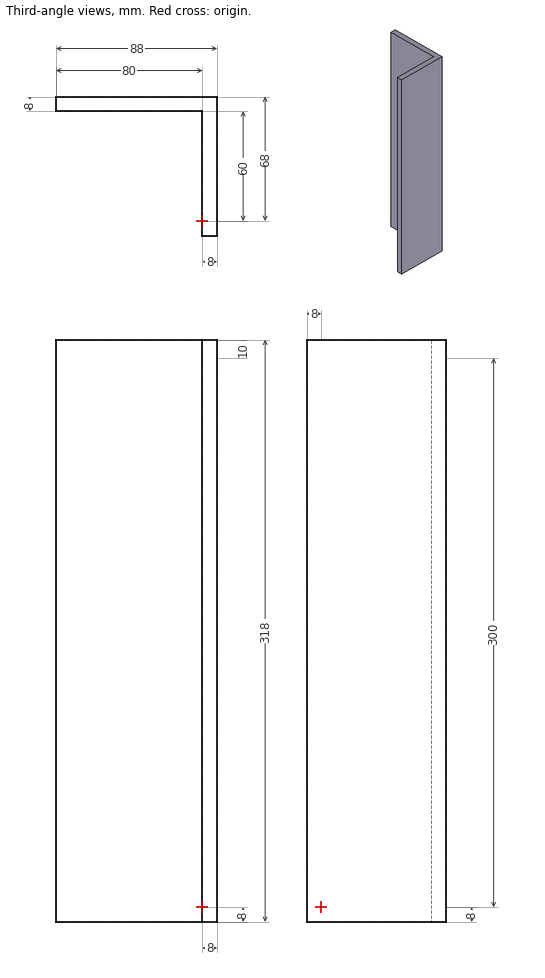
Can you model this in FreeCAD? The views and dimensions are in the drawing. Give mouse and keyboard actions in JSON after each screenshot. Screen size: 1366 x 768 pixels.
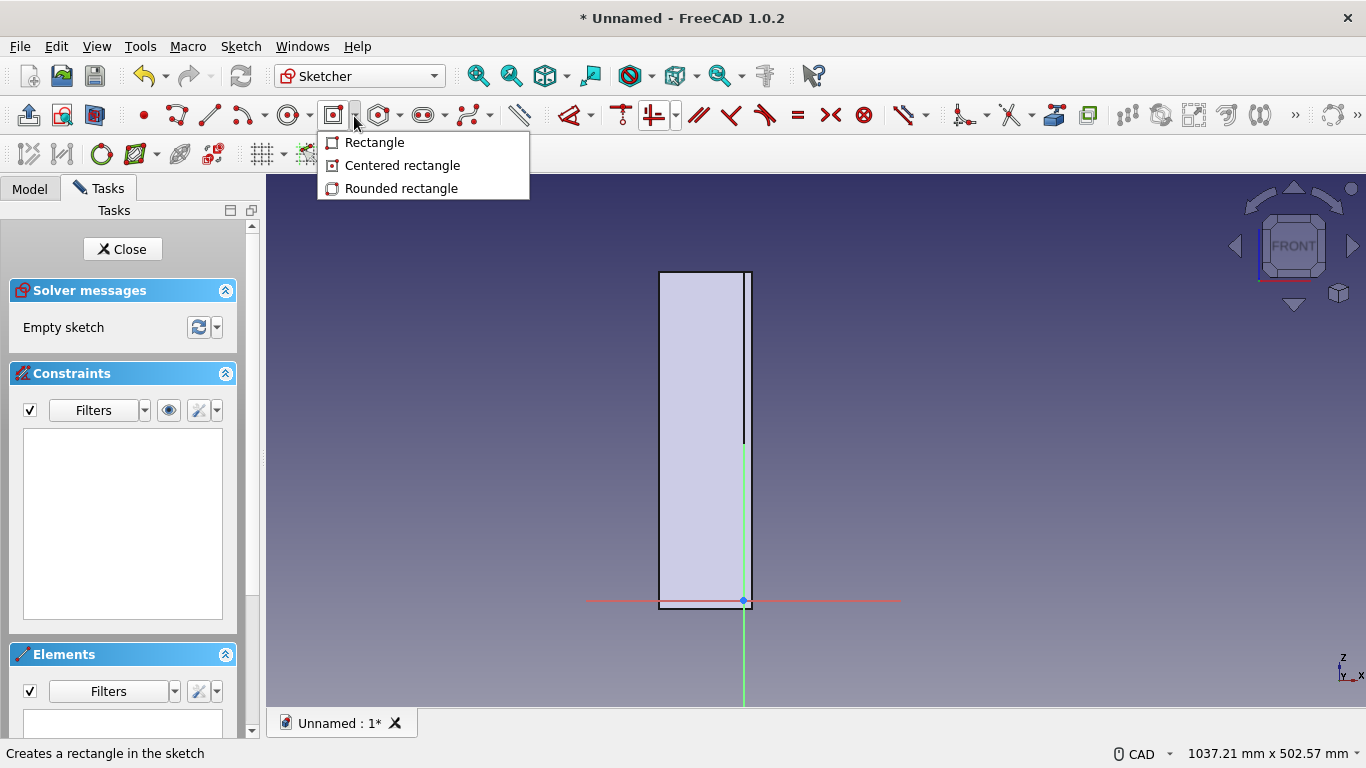
{"action": "left_click", "coordinate": [424, 142]}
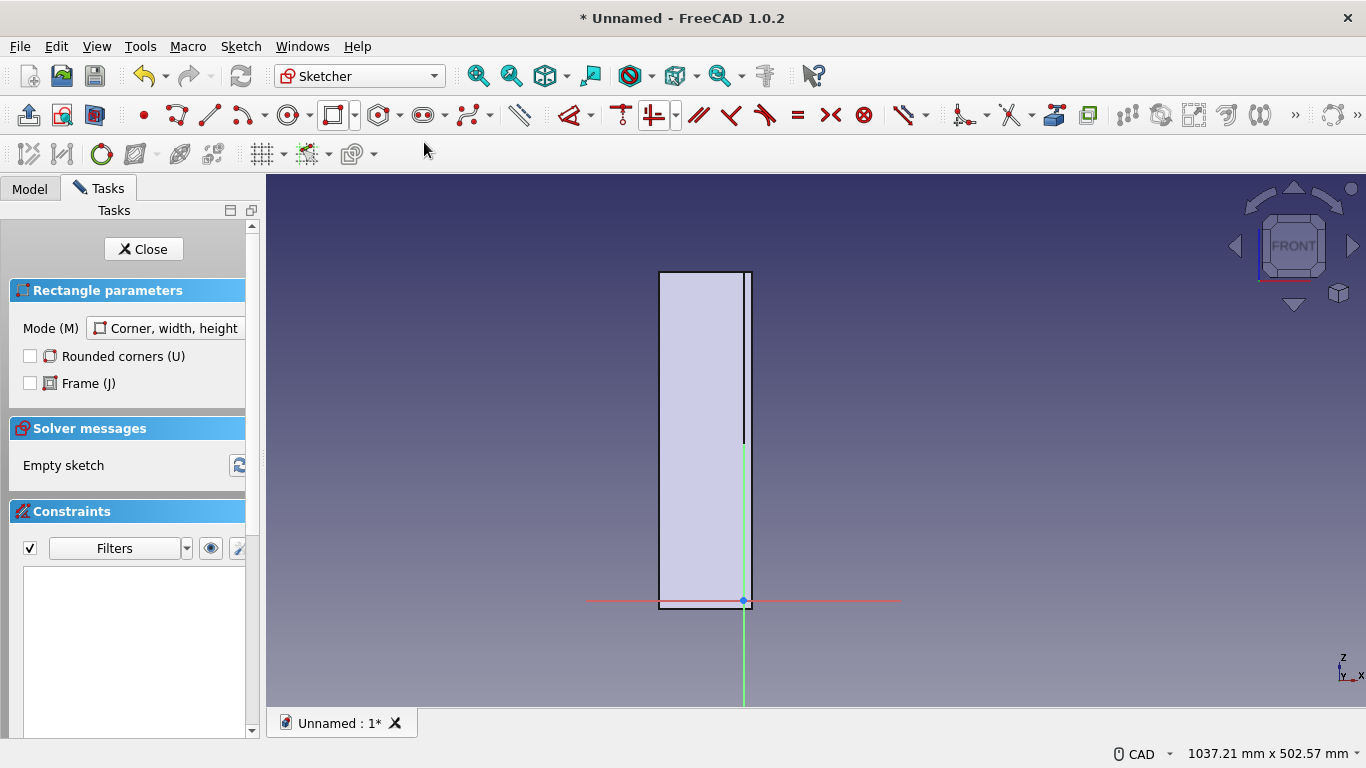
{"action": "scroll", "coordinate": [744, 272], "scroll_direction": "up", "scroll_amount": 4}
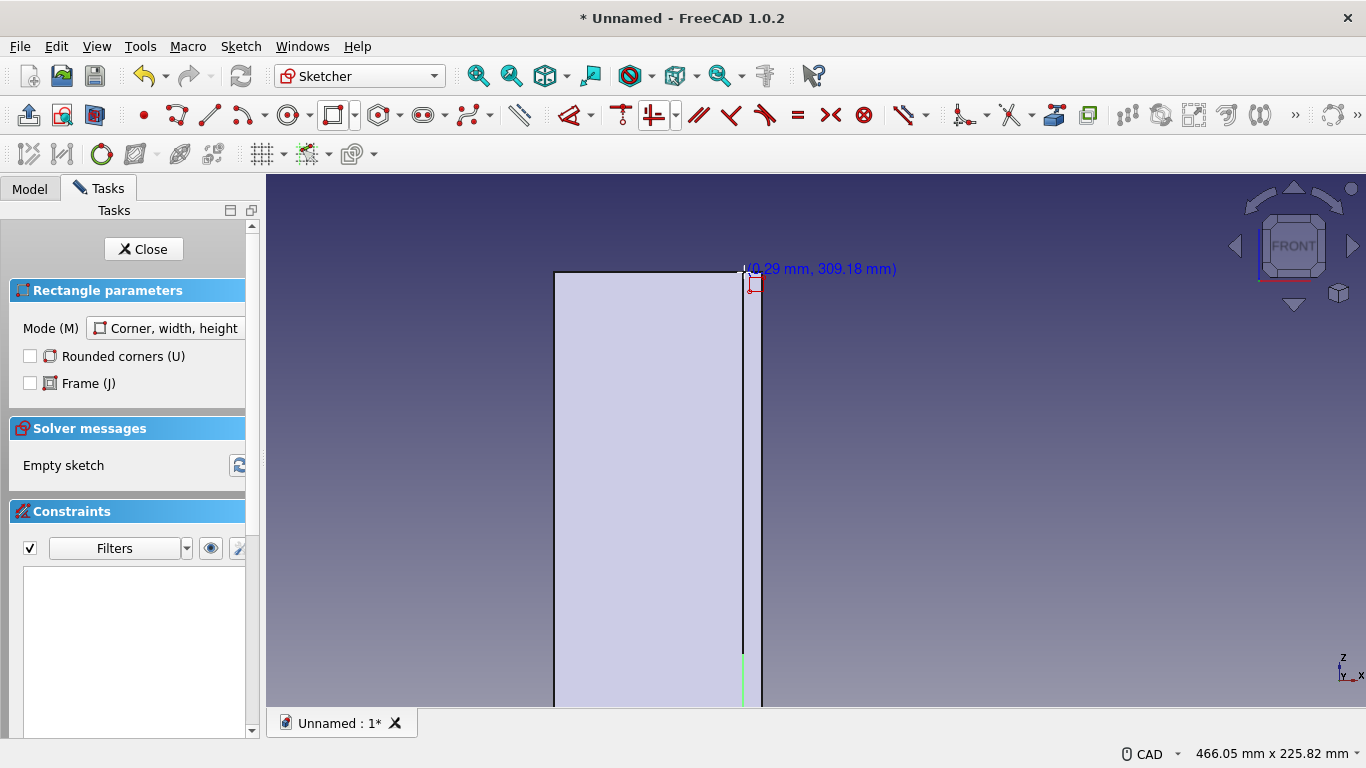
{"action": "left_click", "coordinate": [743, 272]}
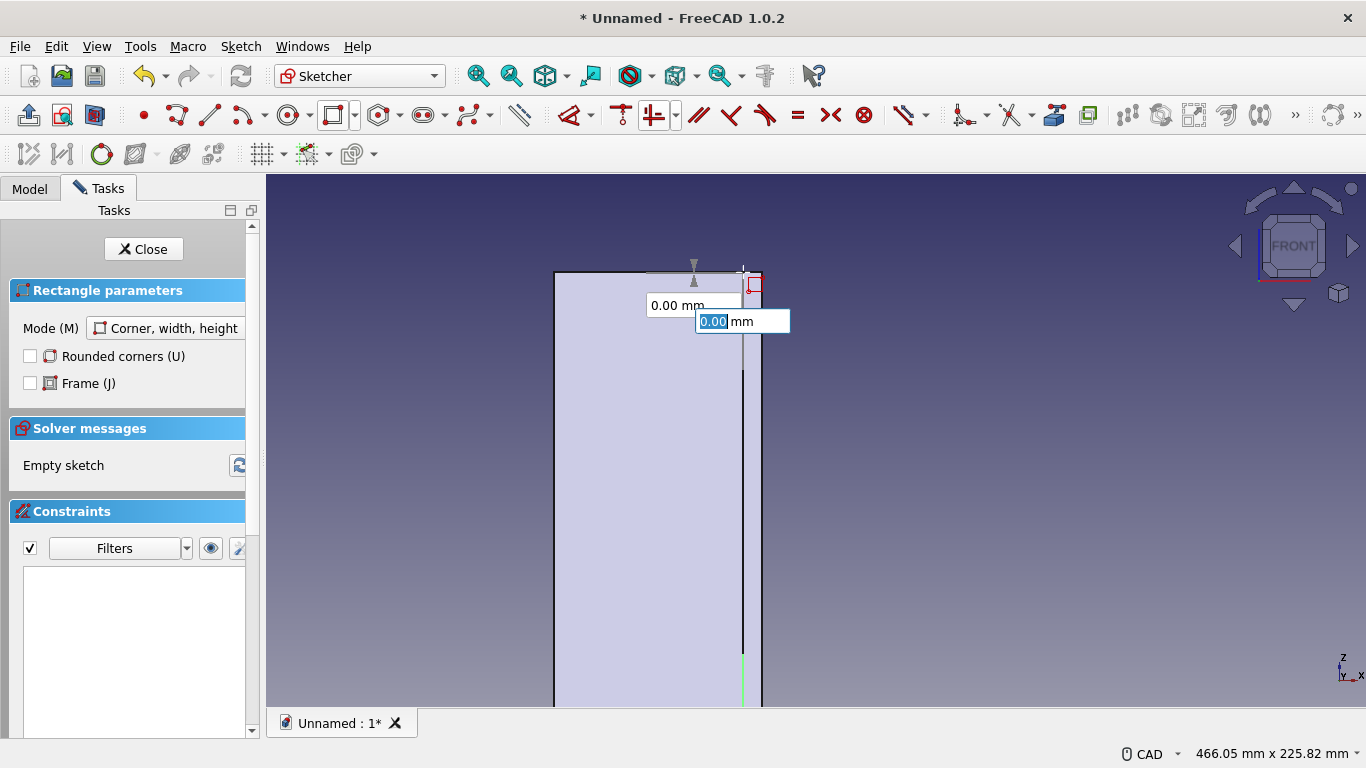
{"action": "scroll", "coordinate": [744, 272], "scroll_direction": "down", "scroll_amount": 4}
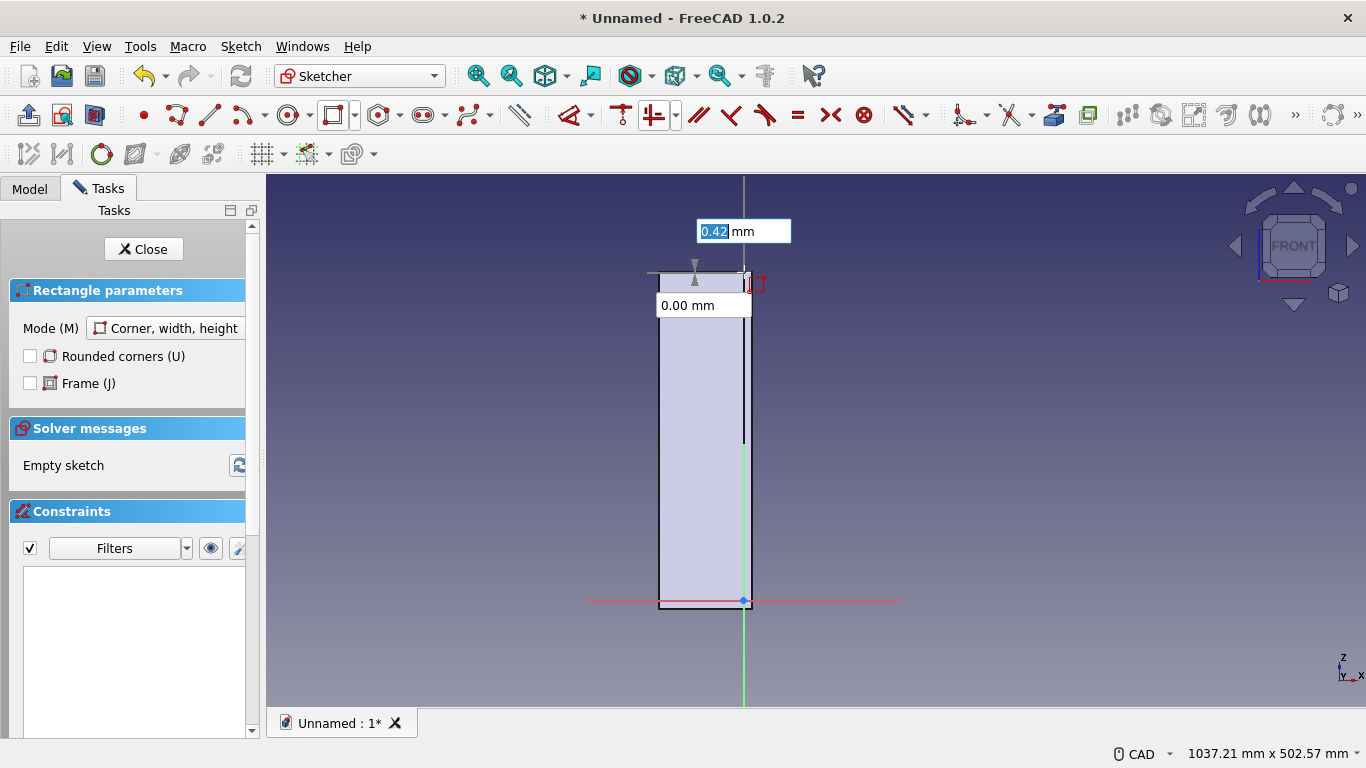
{"action": "scroll", "coordinate": [752, 609], "scroll_direction": "up", "scroll_amount": 4}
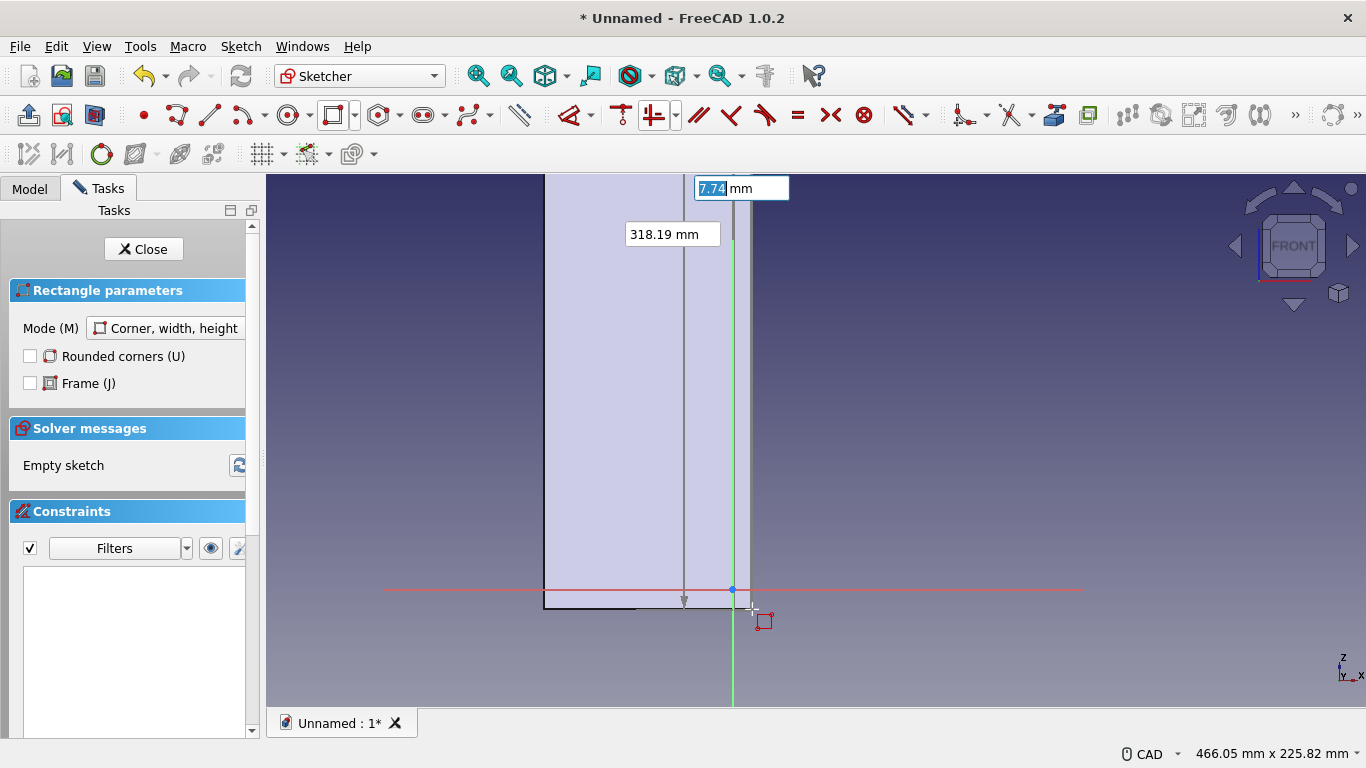
{"action": "left_click", "coordinate": [752, 609]}
{"action": "key", "text": "Escape"}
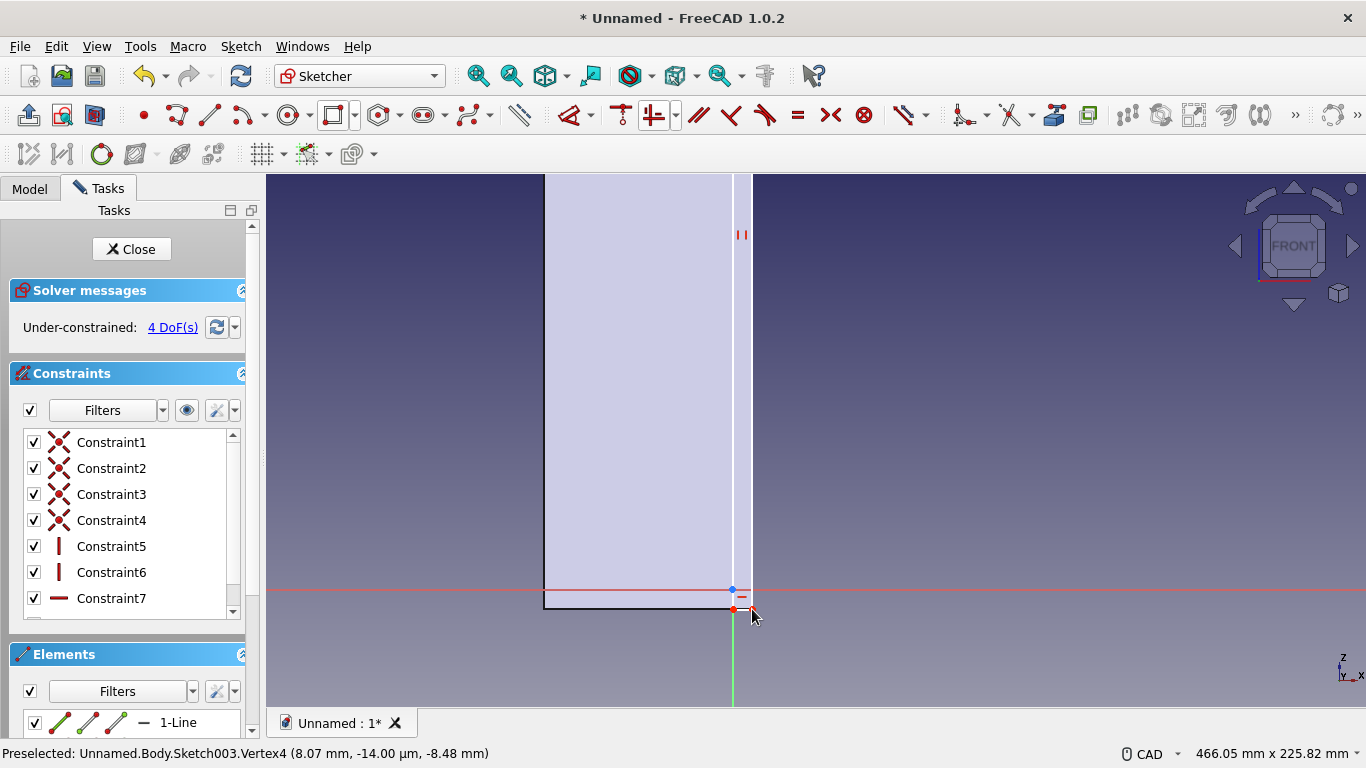
{"action": "scroll", "coordinate": [752, 609], "scroll_direction": "down", "scroll_amount": 4}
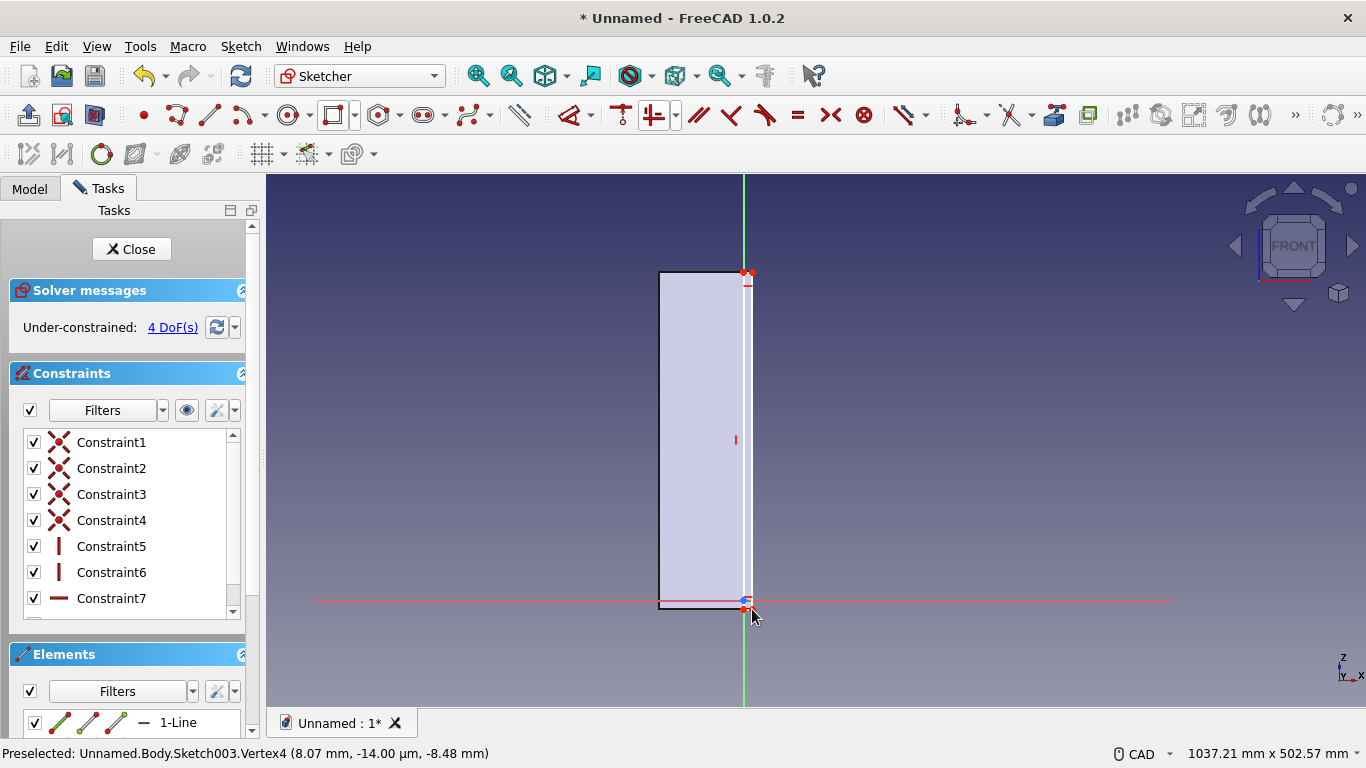
{"action": "scroll", "coordinate": [744, 273], "scroll_direction": "up", "scroll_amount": 2}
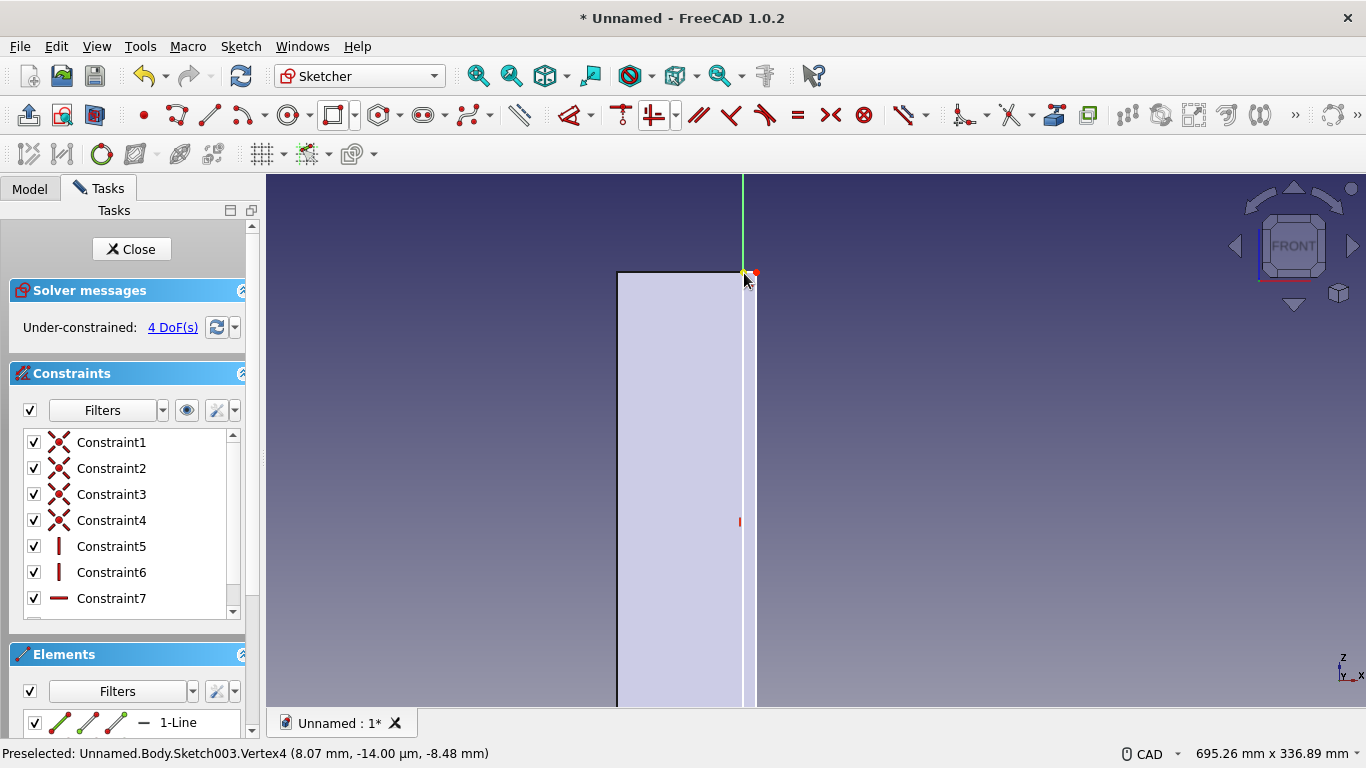
{"action": "left_click", "coordinate": [743, 272]}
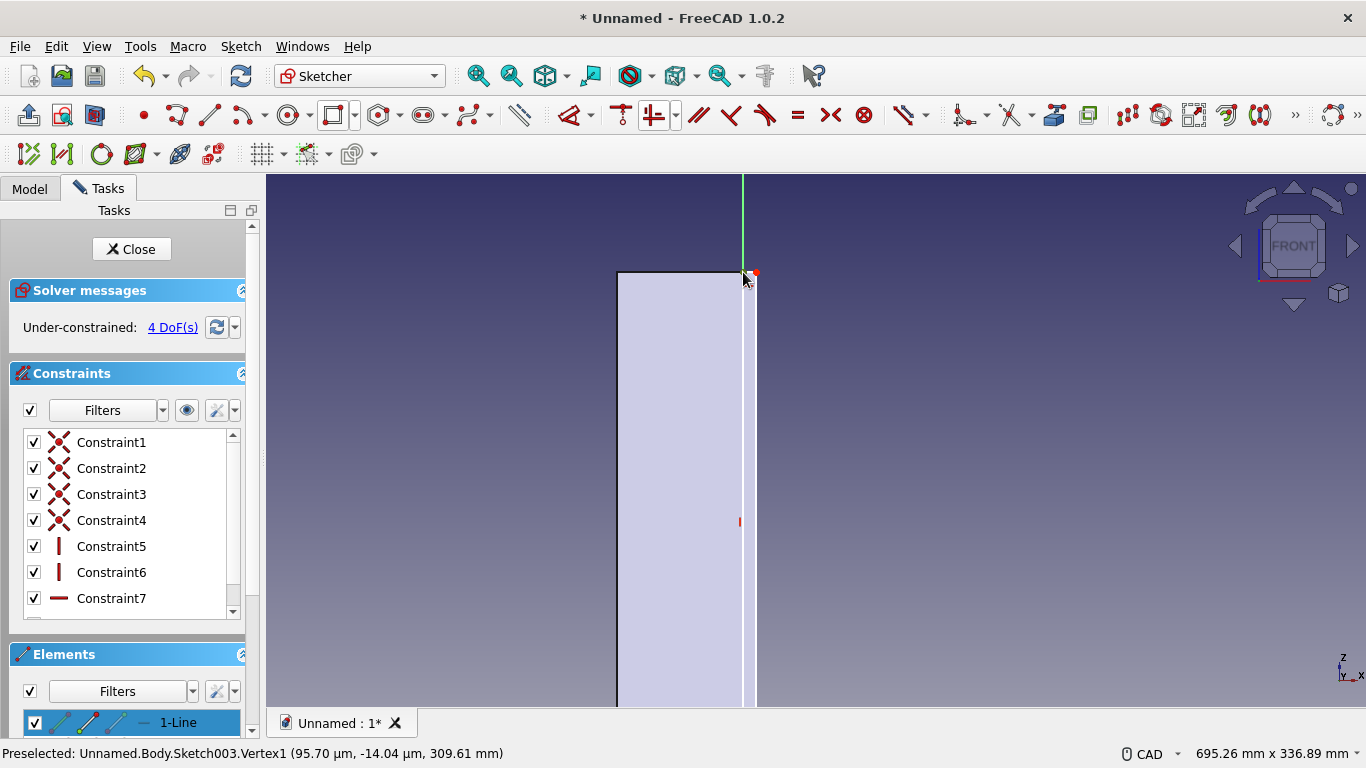
{"action": "left_click", "coordinate": [743, 236]}